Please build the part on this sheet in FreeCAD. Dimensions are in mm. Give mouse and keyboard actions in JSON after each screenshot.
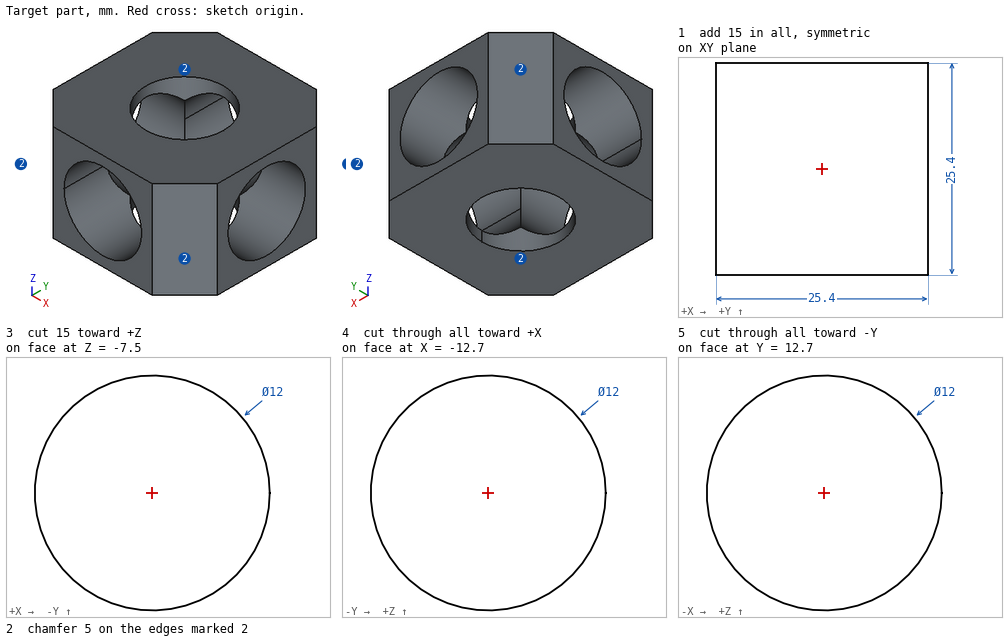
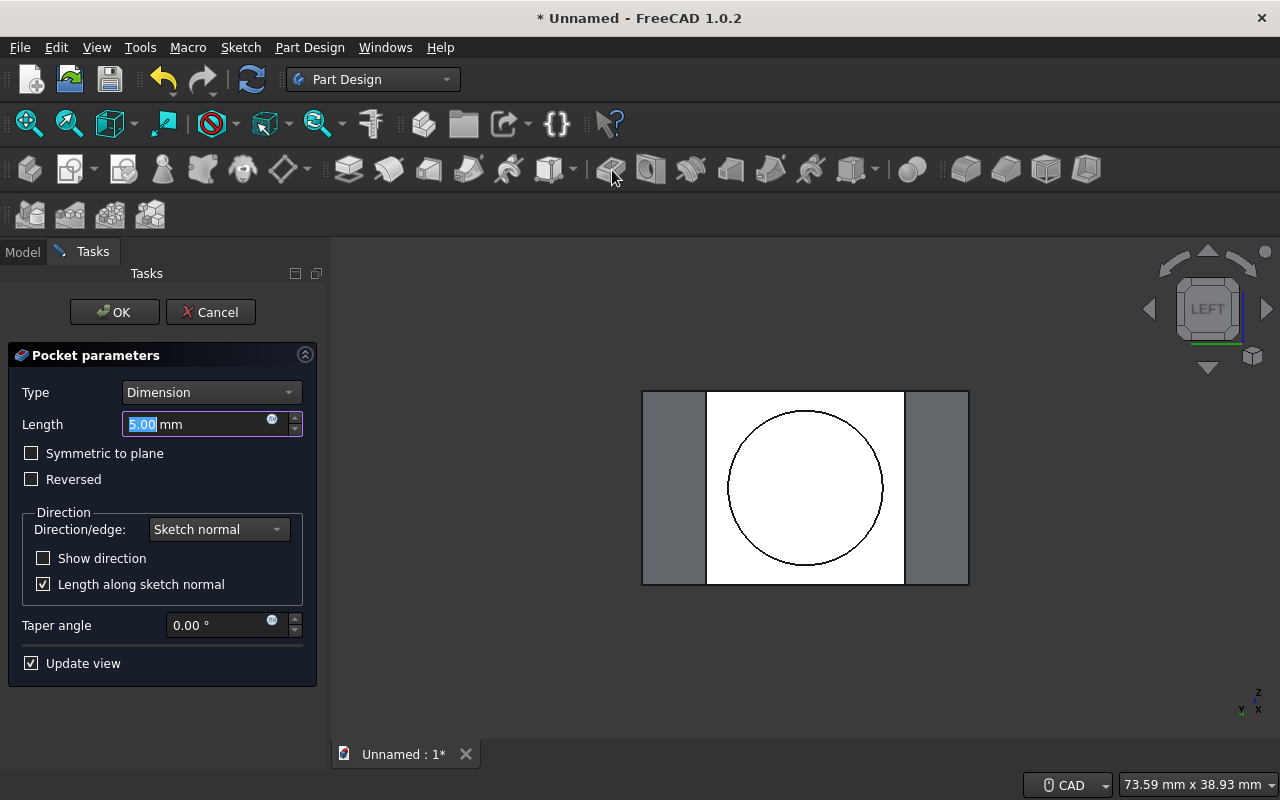
{"action": "left_click", "coordinate": [212, 392]}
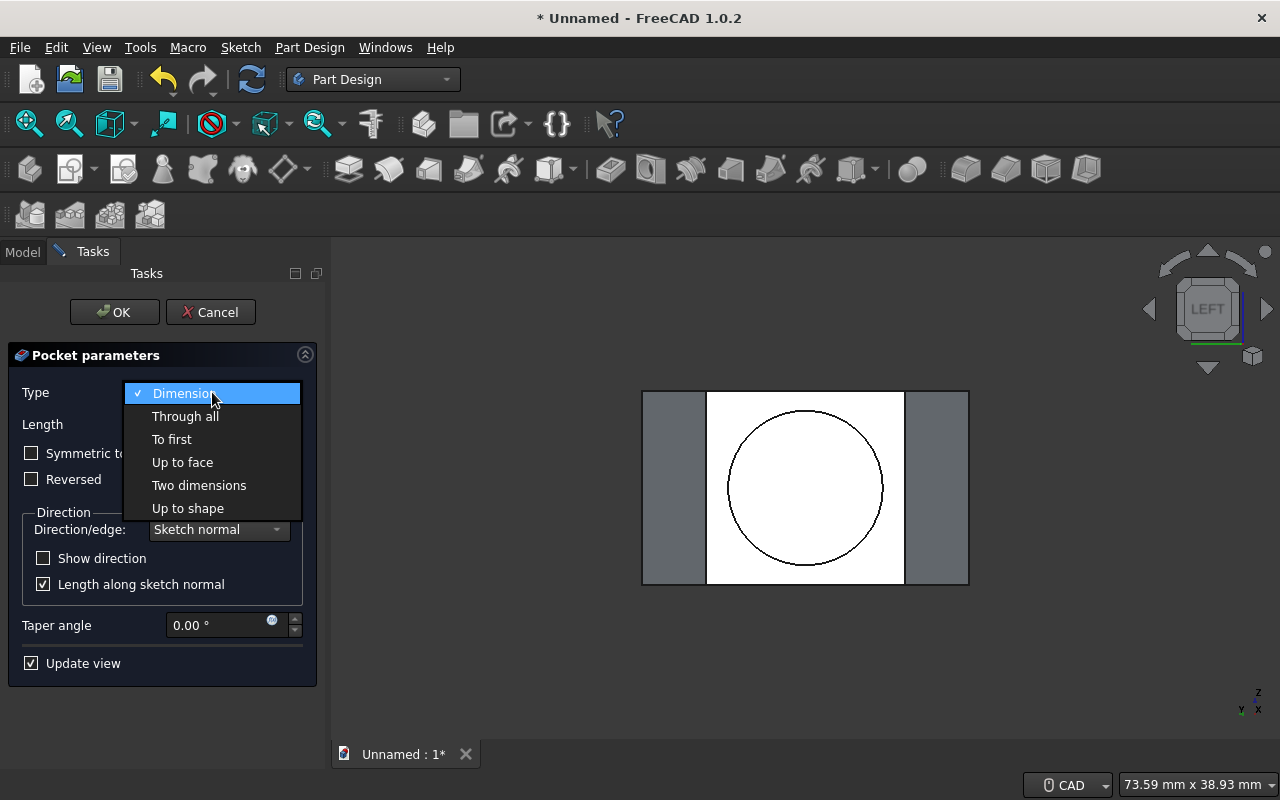
{"action": "left_click", "coordinate": [212, 416]}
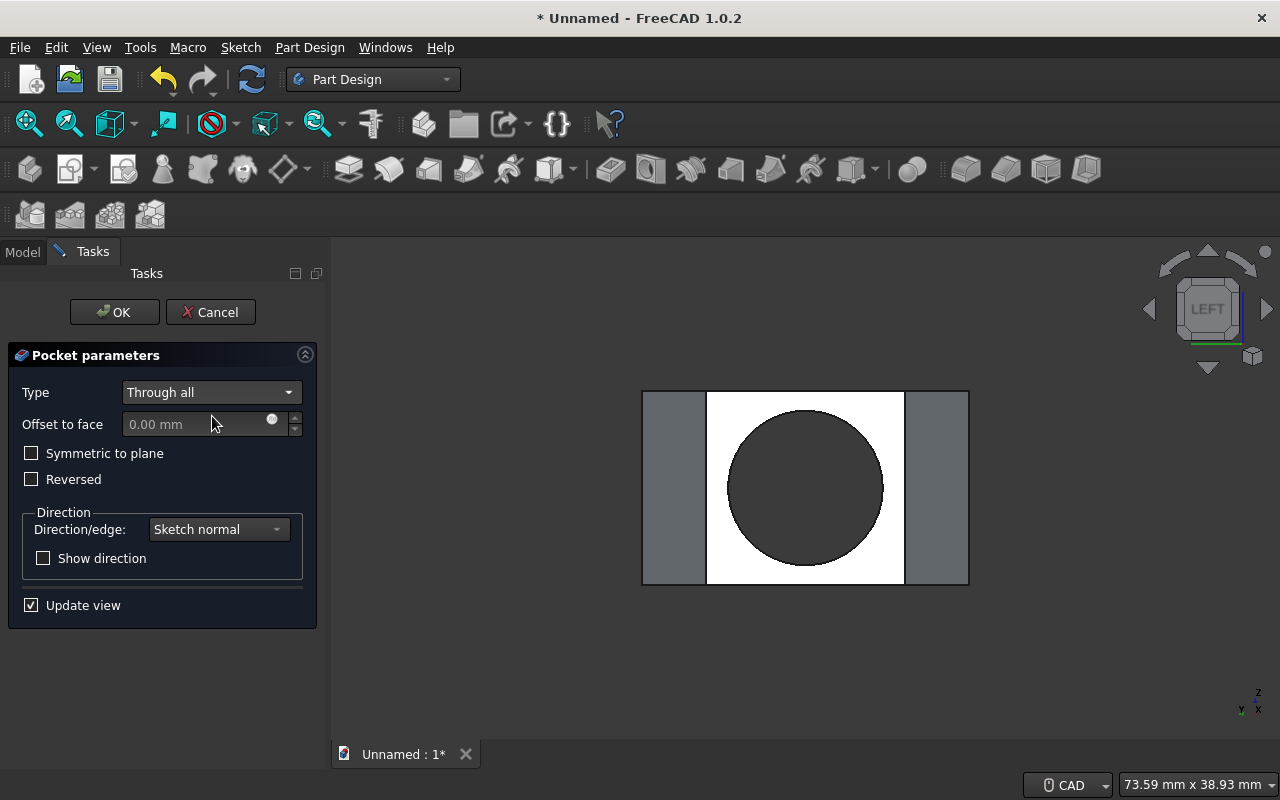
{"action": "left_click", "coordinate": [115, 312]}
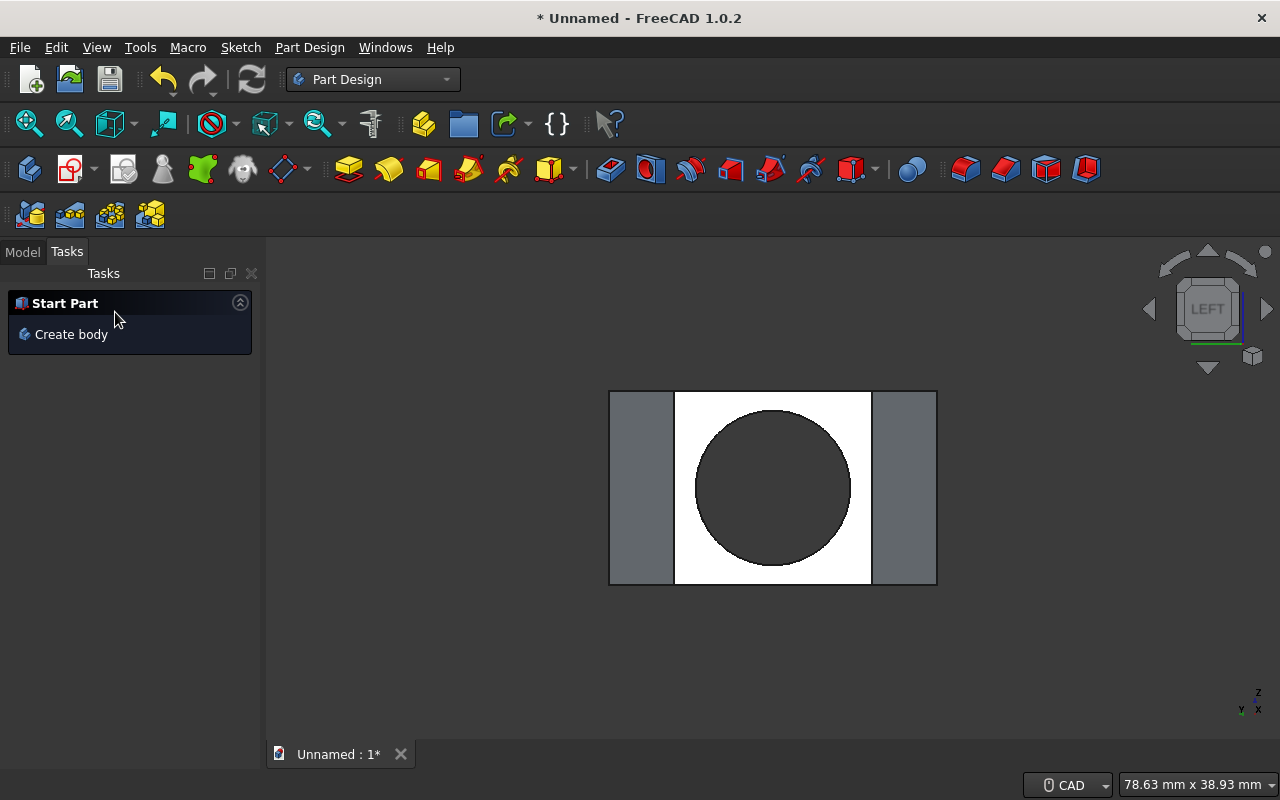
{"action": "key", "text": "v f"}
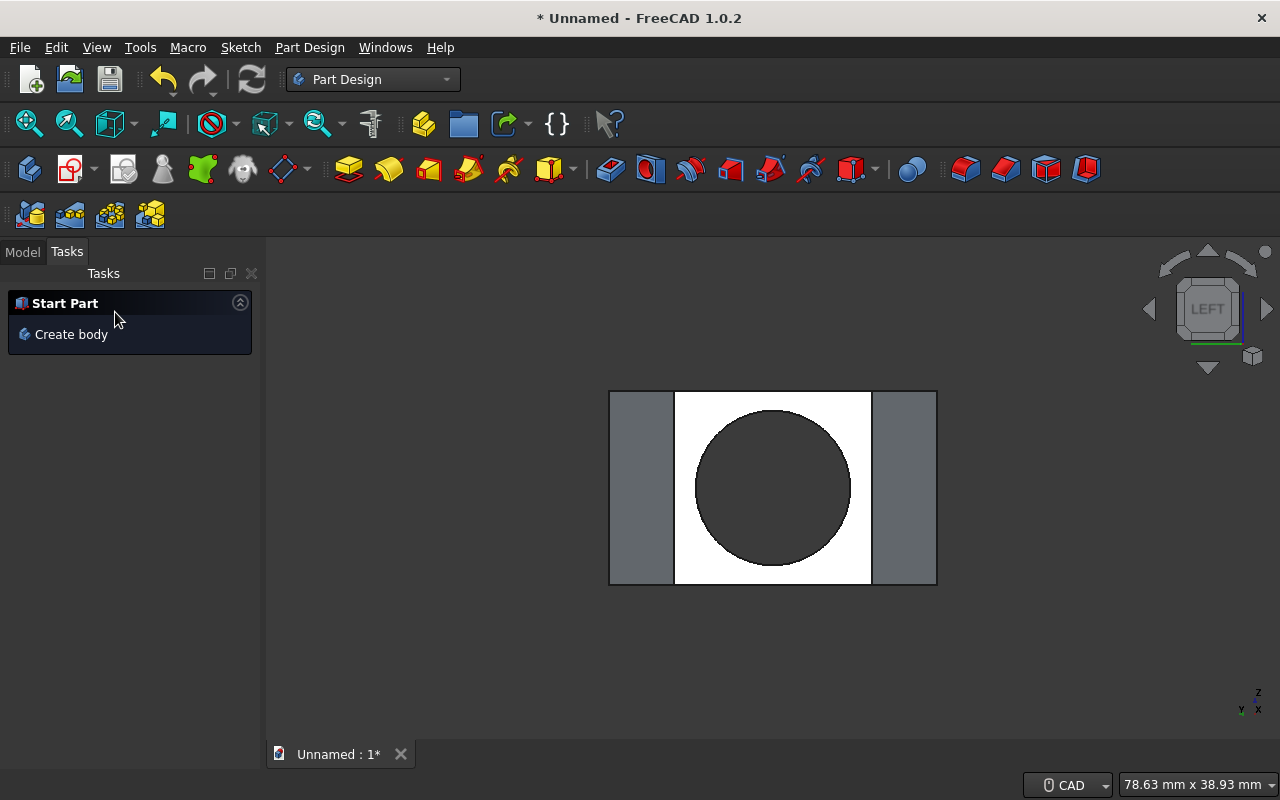
{"action": "key", "text": "4"}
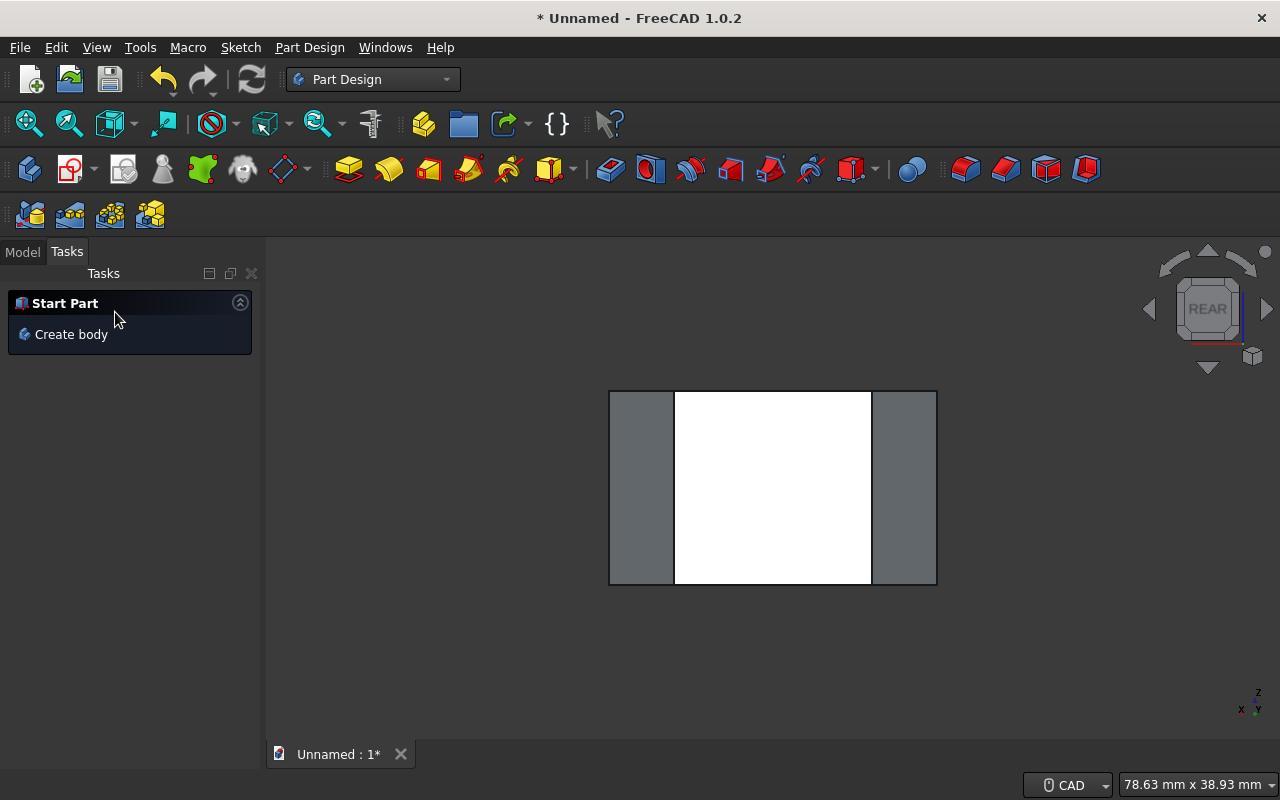
{"action": "key", "text": "v f"}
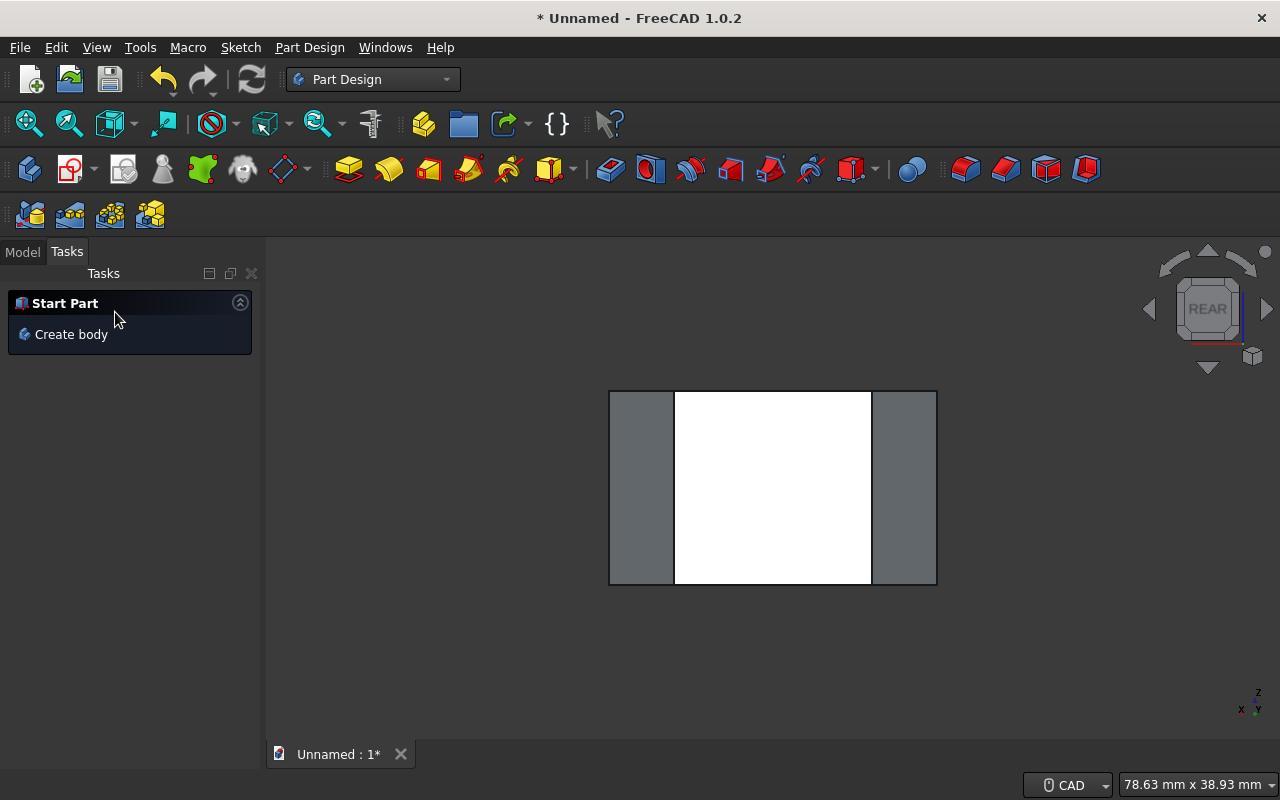
{"action": "left_click", "coordinate": [773, 487]}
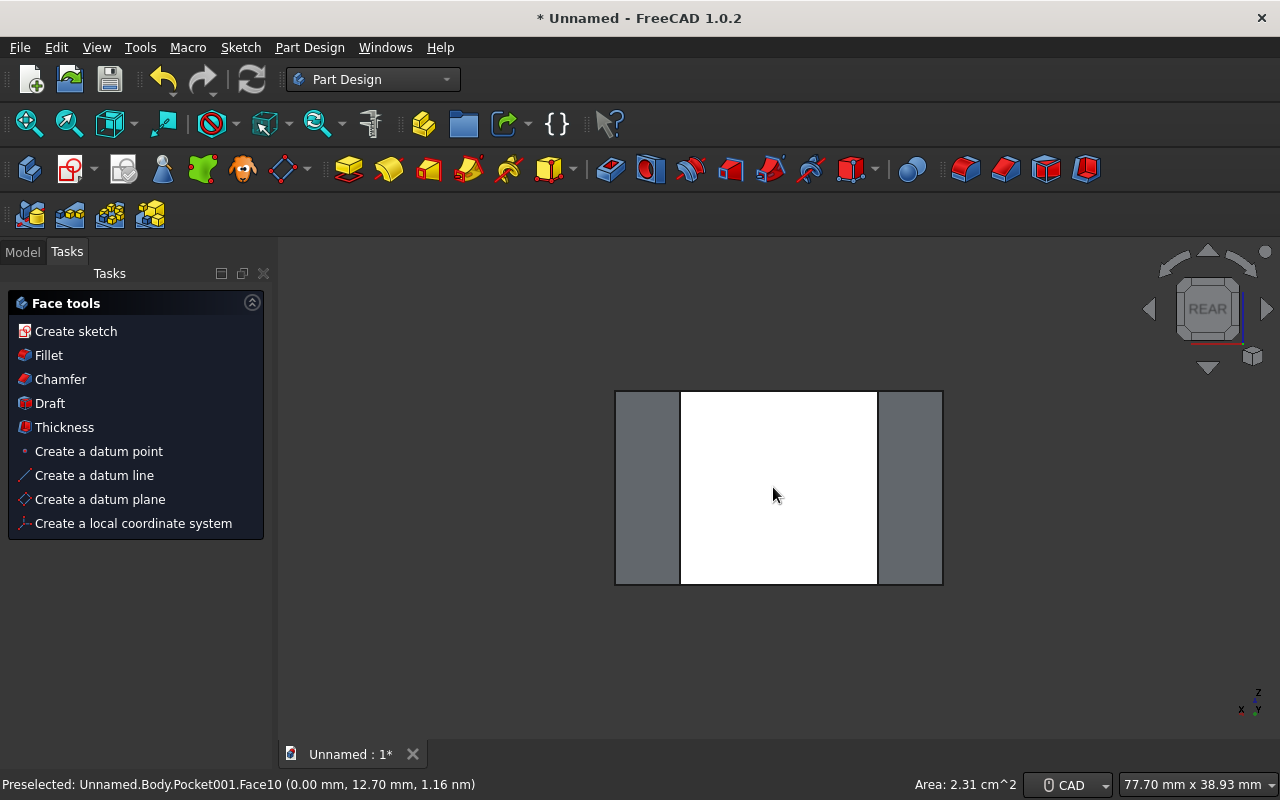
{"action": "left_click", "coordinate": [70, 170]}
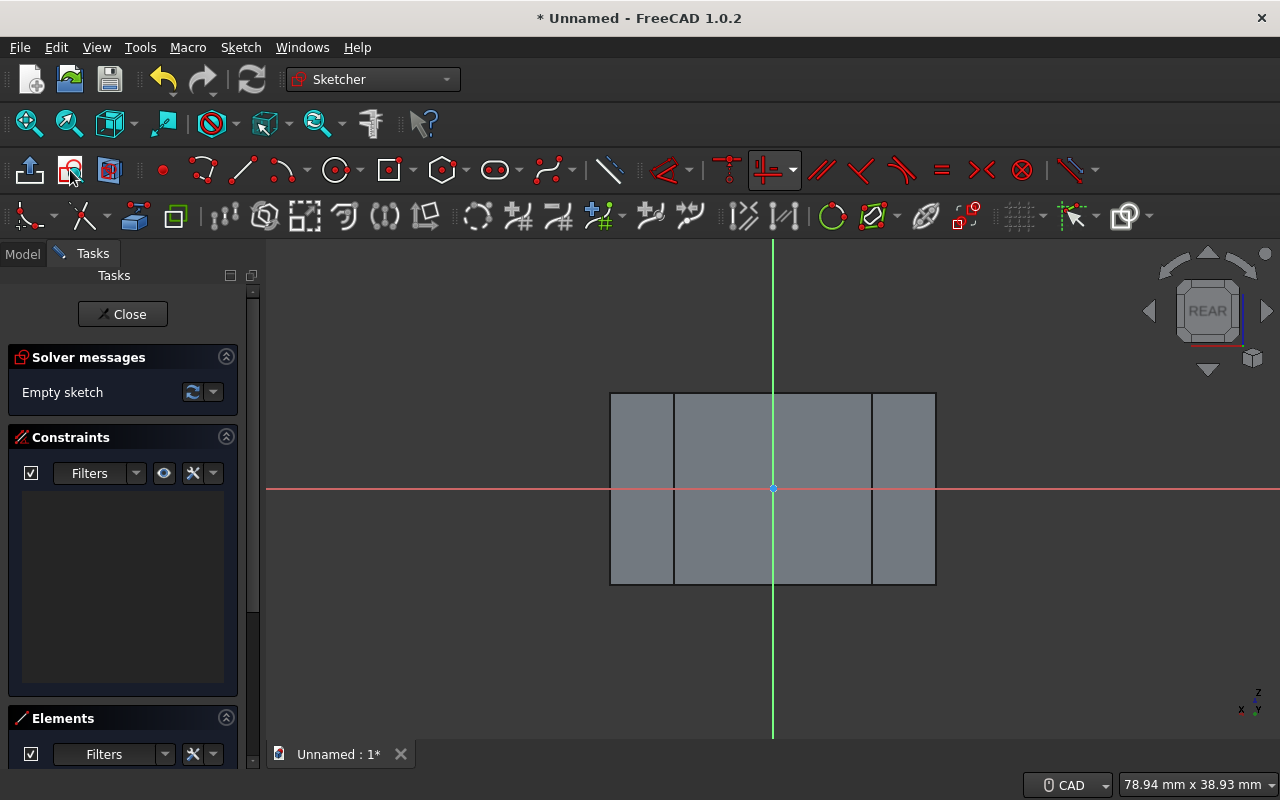
{"action": "scroll", "coordinate": [829, 489], "scroll_direction": "up", "scroll_amount": 4}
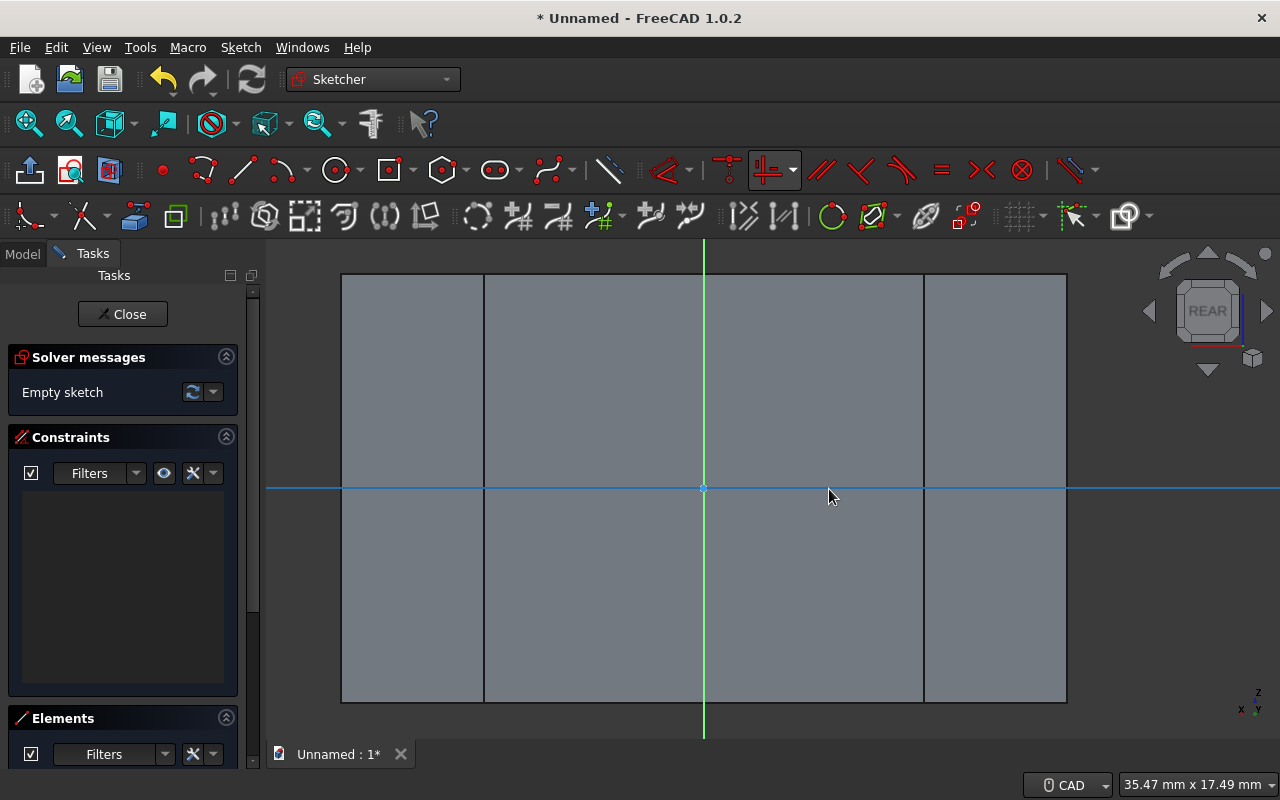
{"action": "key", "text": "g c"}